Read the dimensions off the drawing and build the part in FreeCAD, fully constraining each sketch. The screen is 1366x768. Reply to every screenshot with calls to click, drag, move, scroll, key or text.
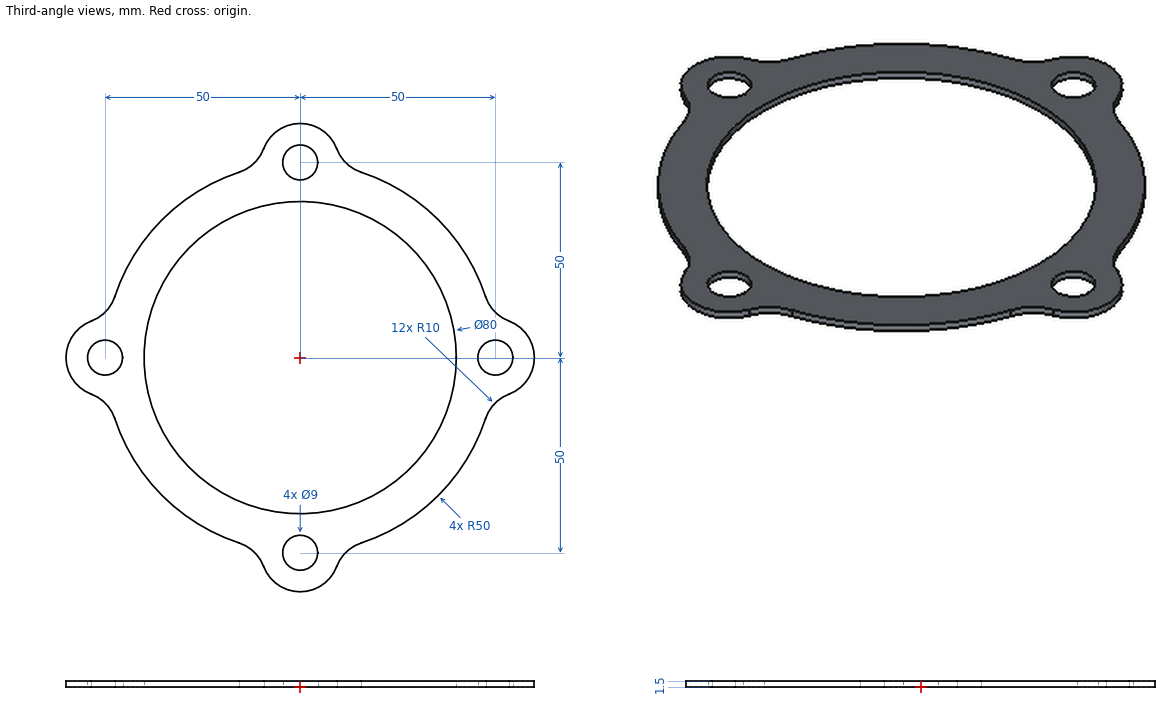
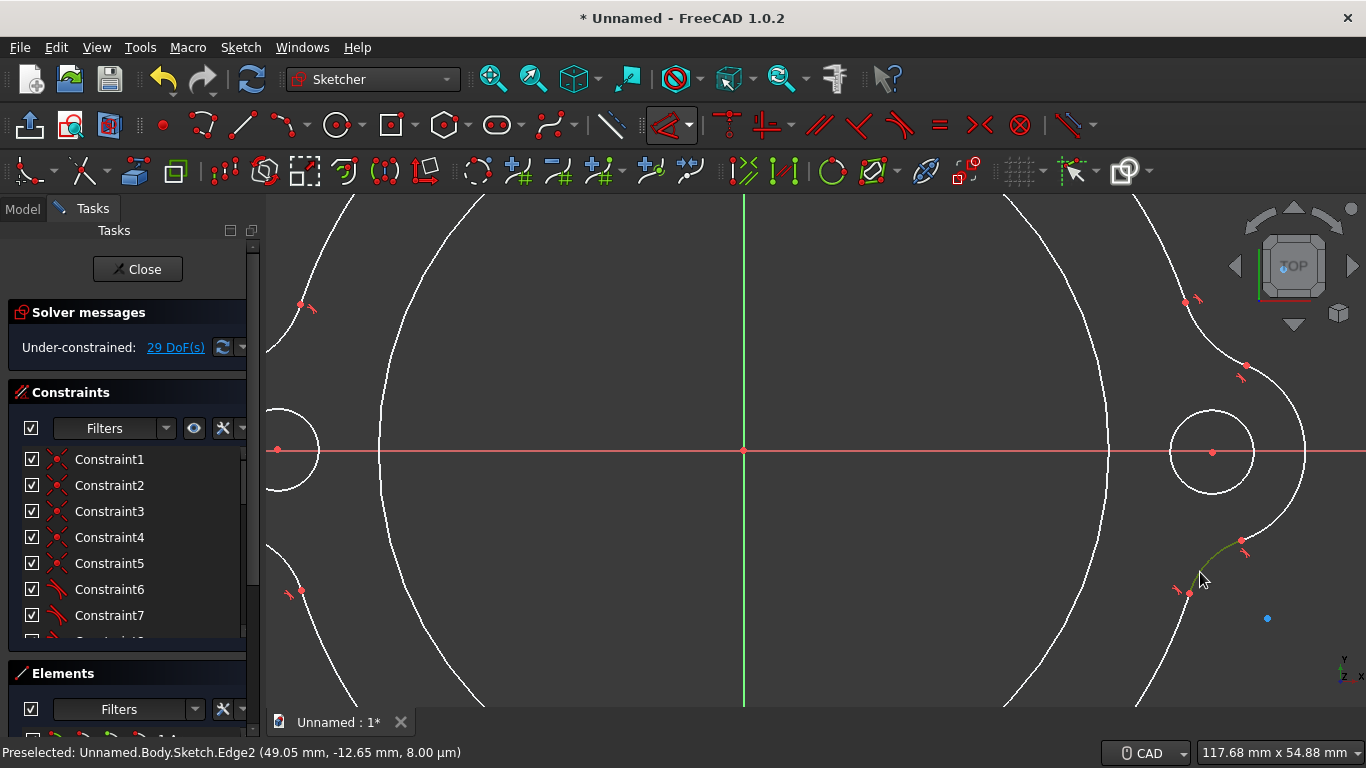
scroll(749, 450, down, 6)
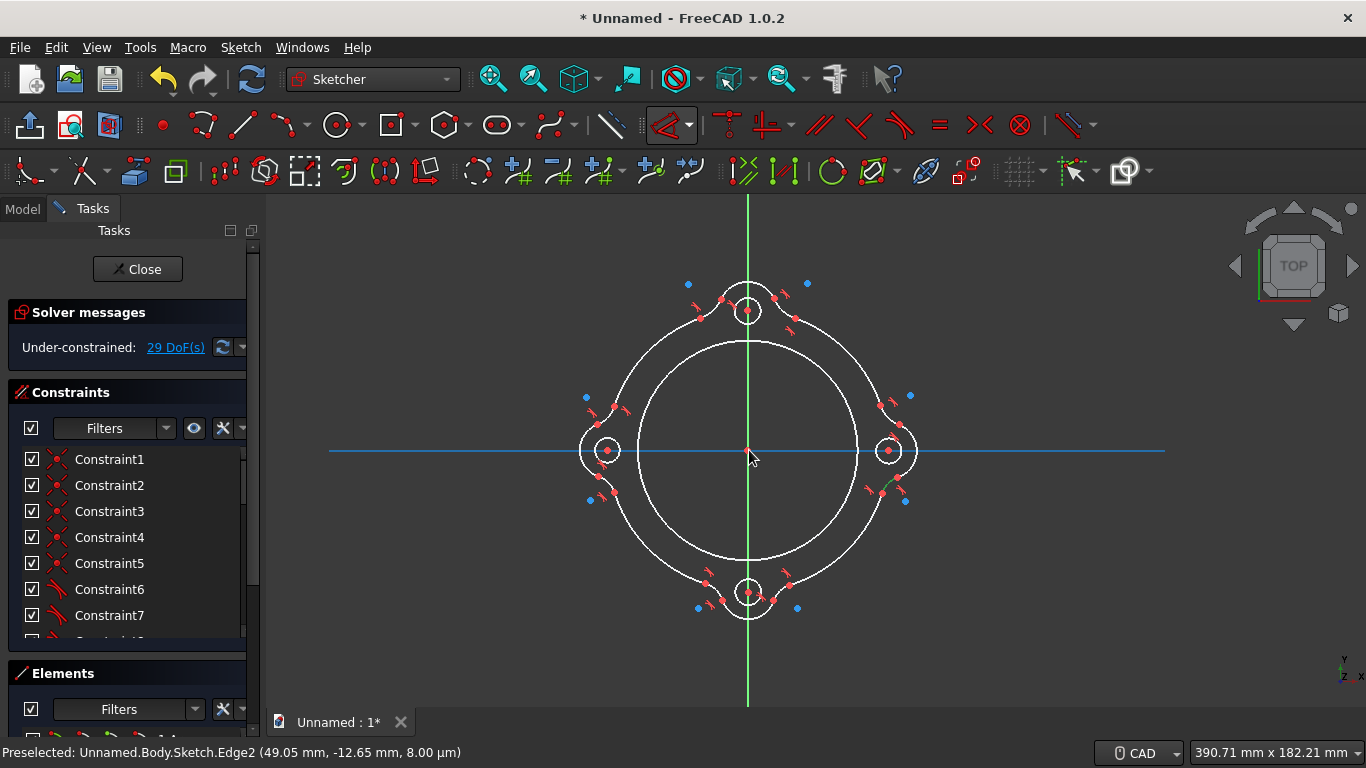
click(913, 465)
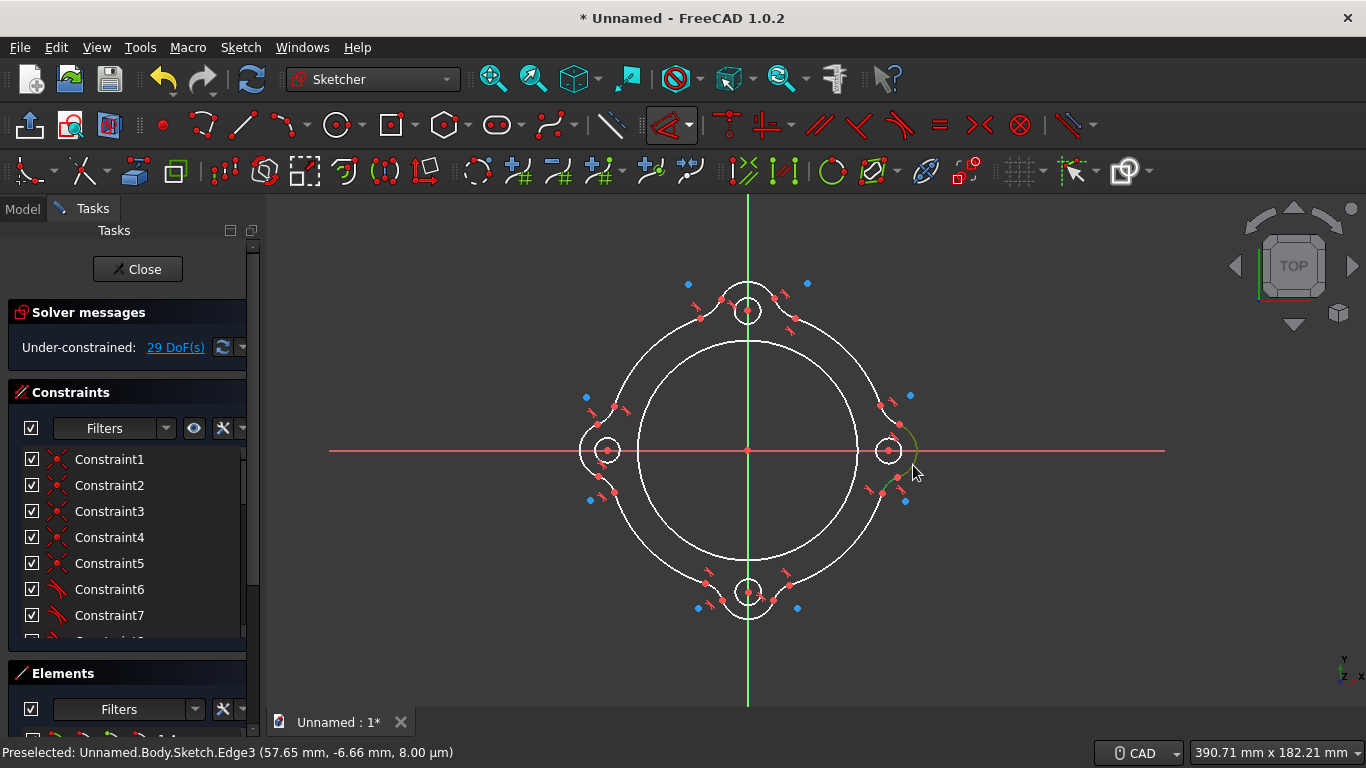
click(888, 417)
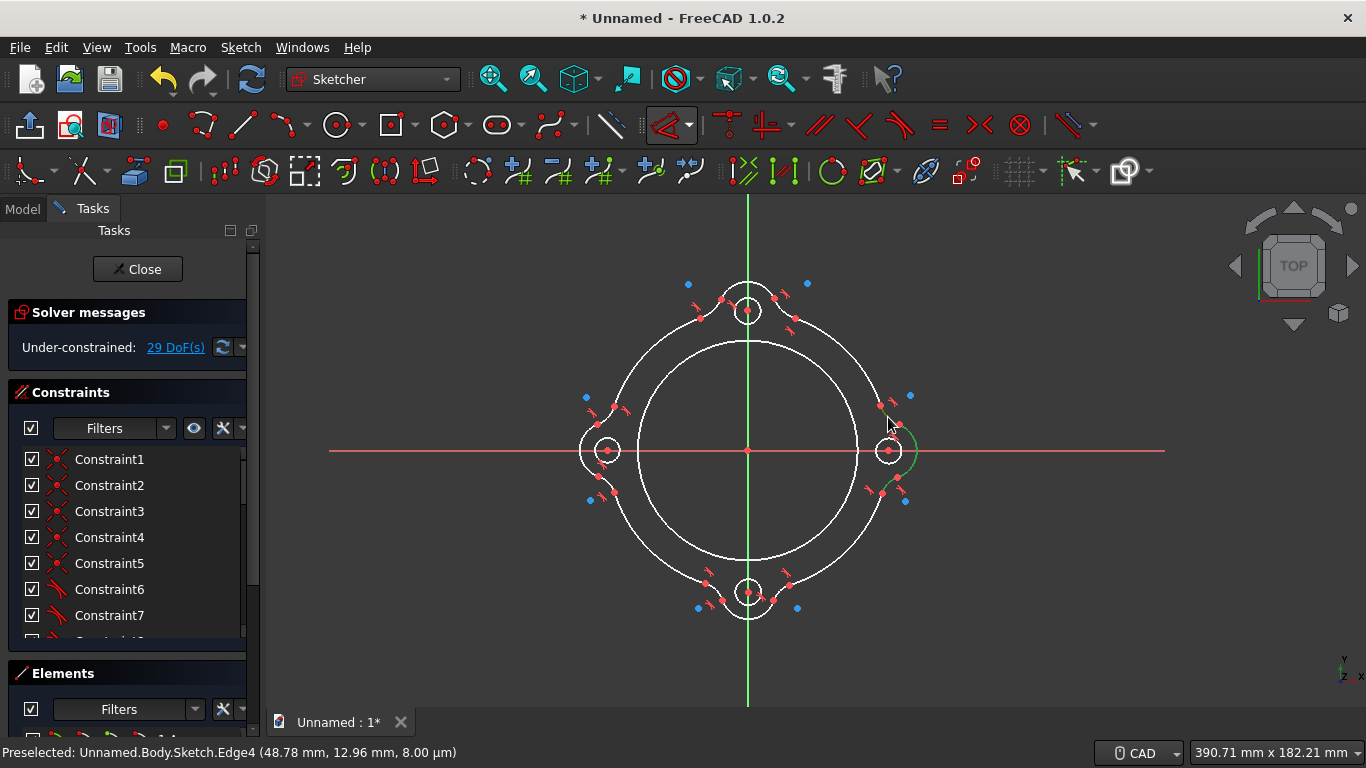
click(783, 311)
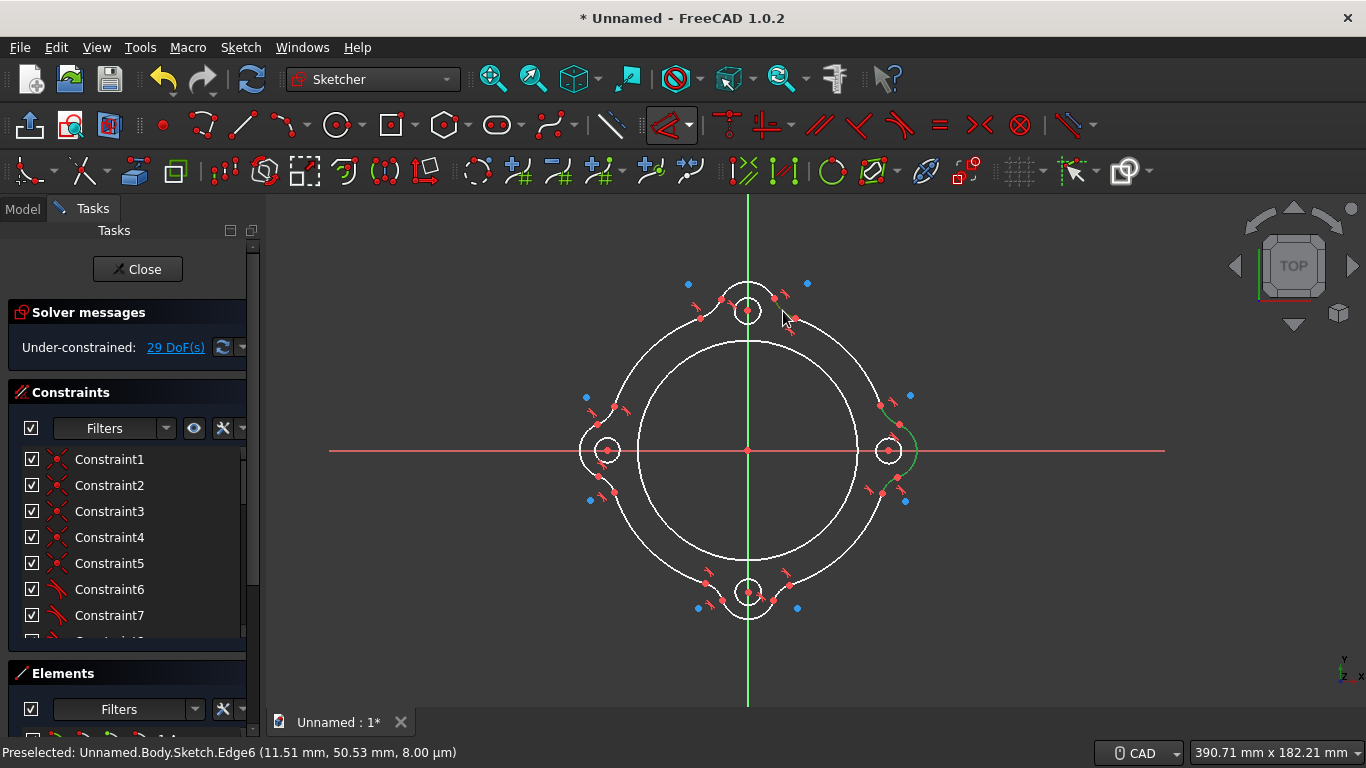
click(760, 285)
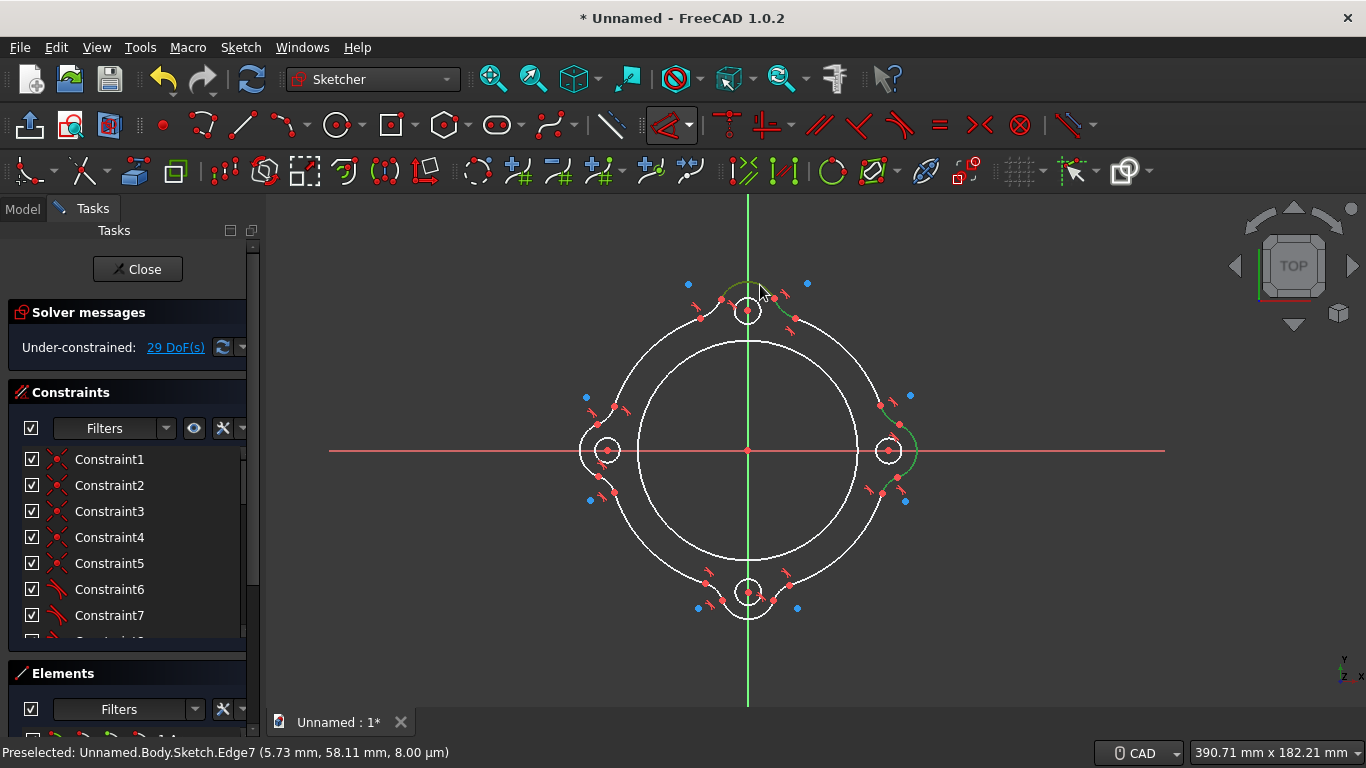
click(713, 311)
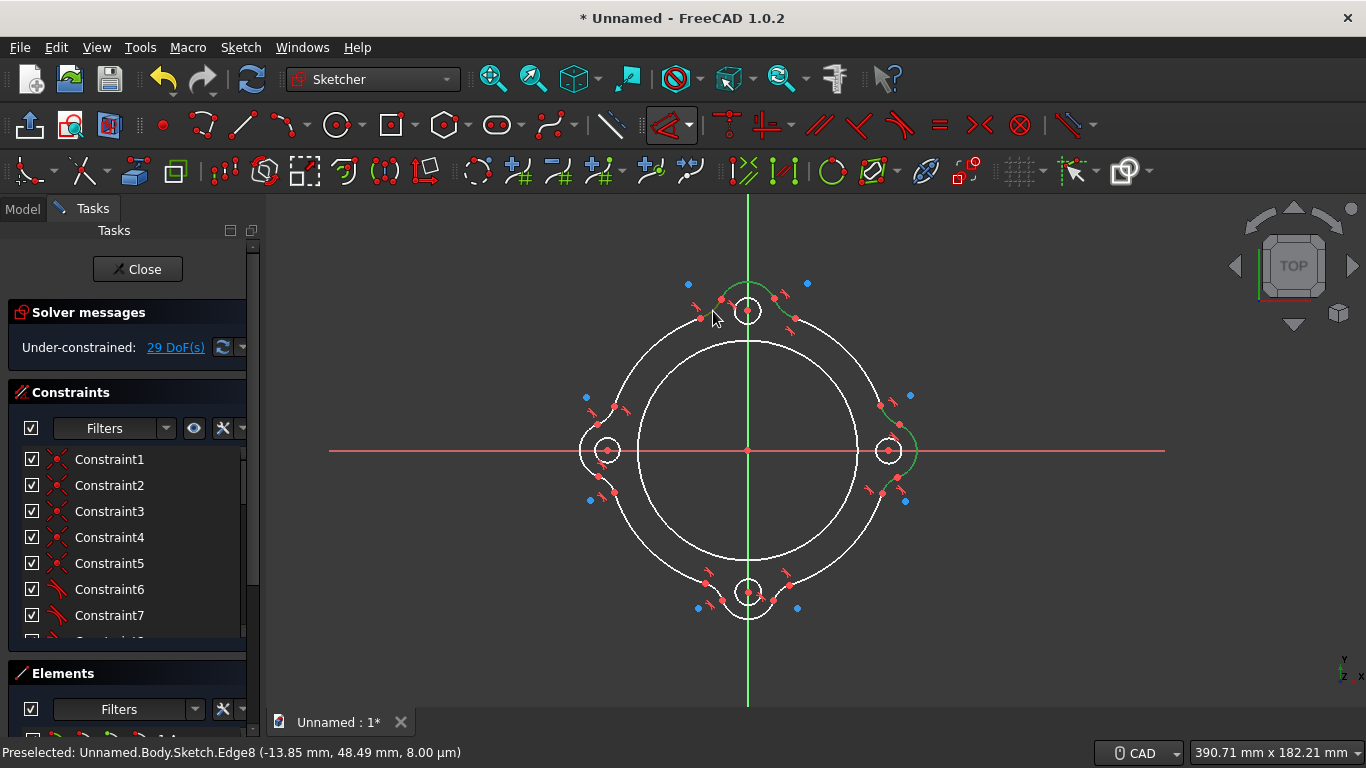
click(608, 418)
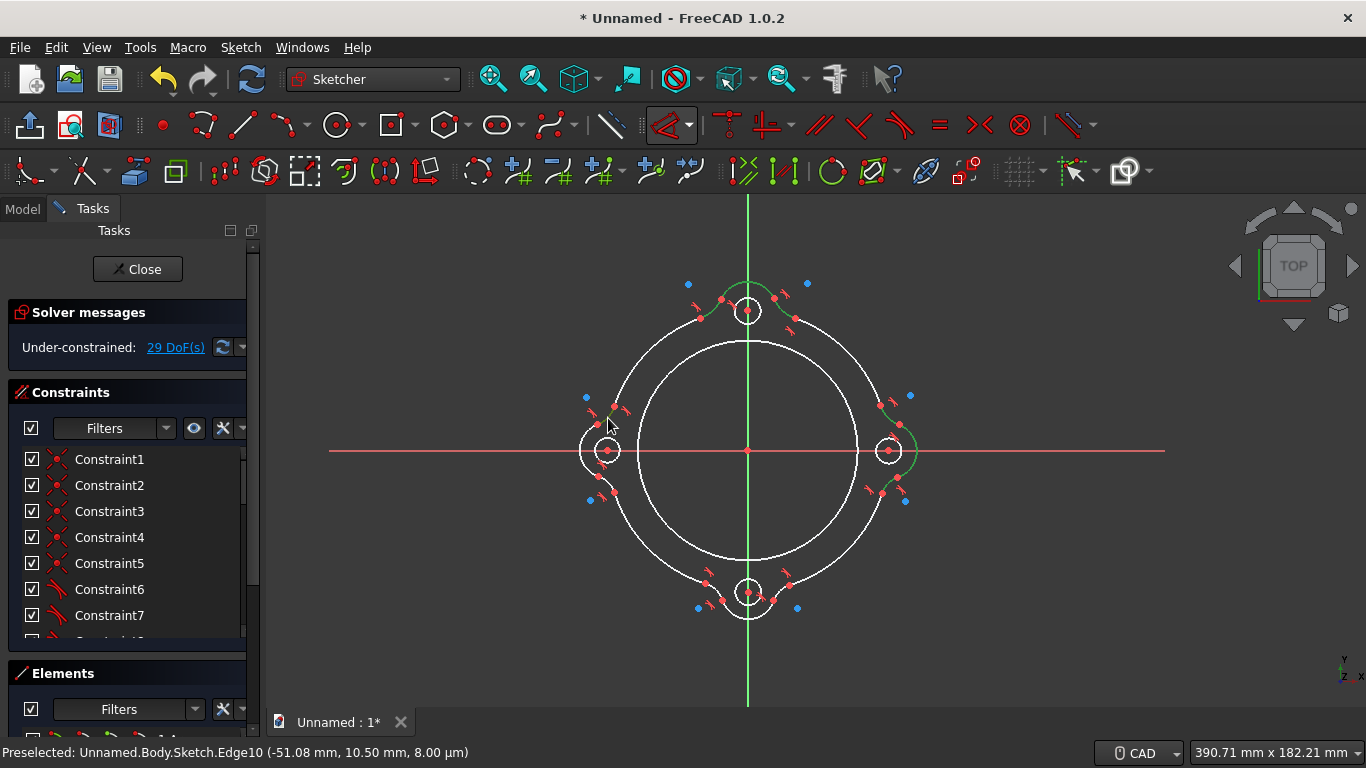
click(583, 438)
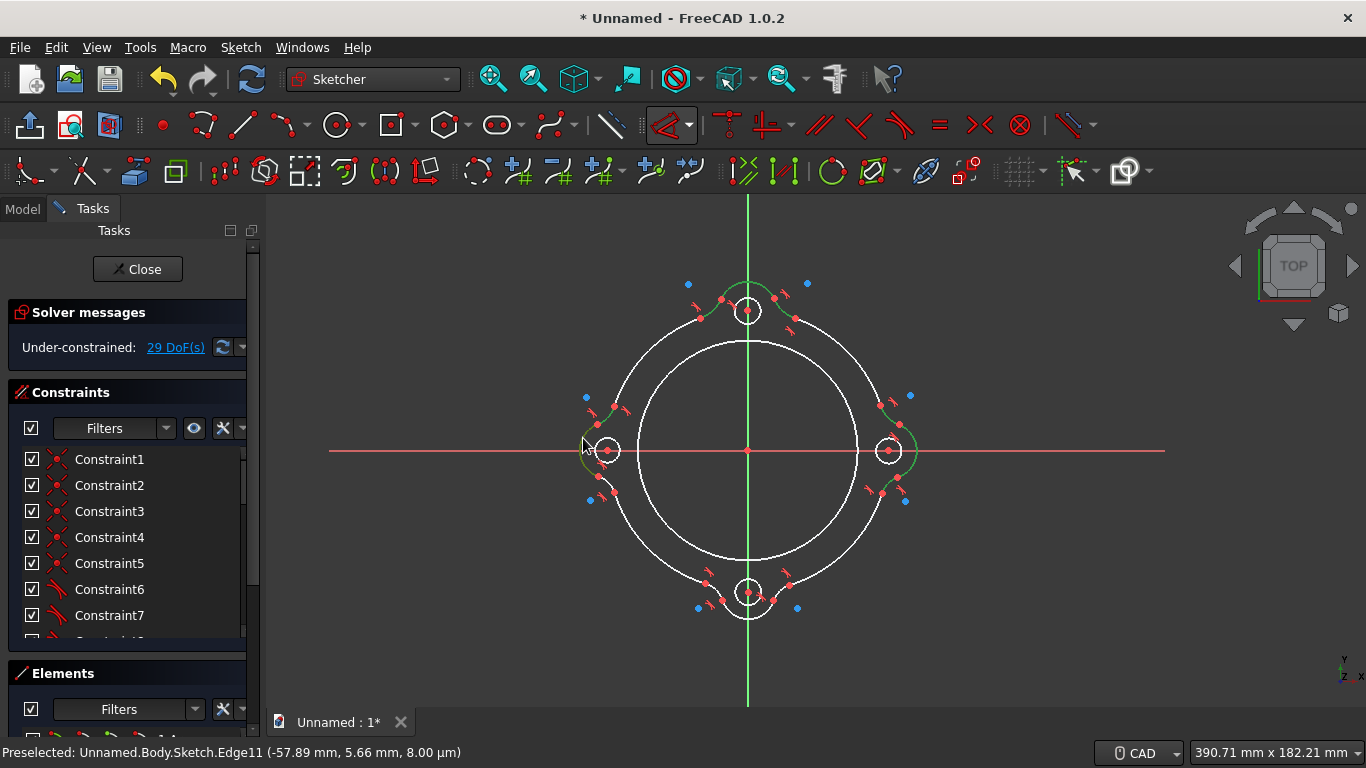
click(608, 483)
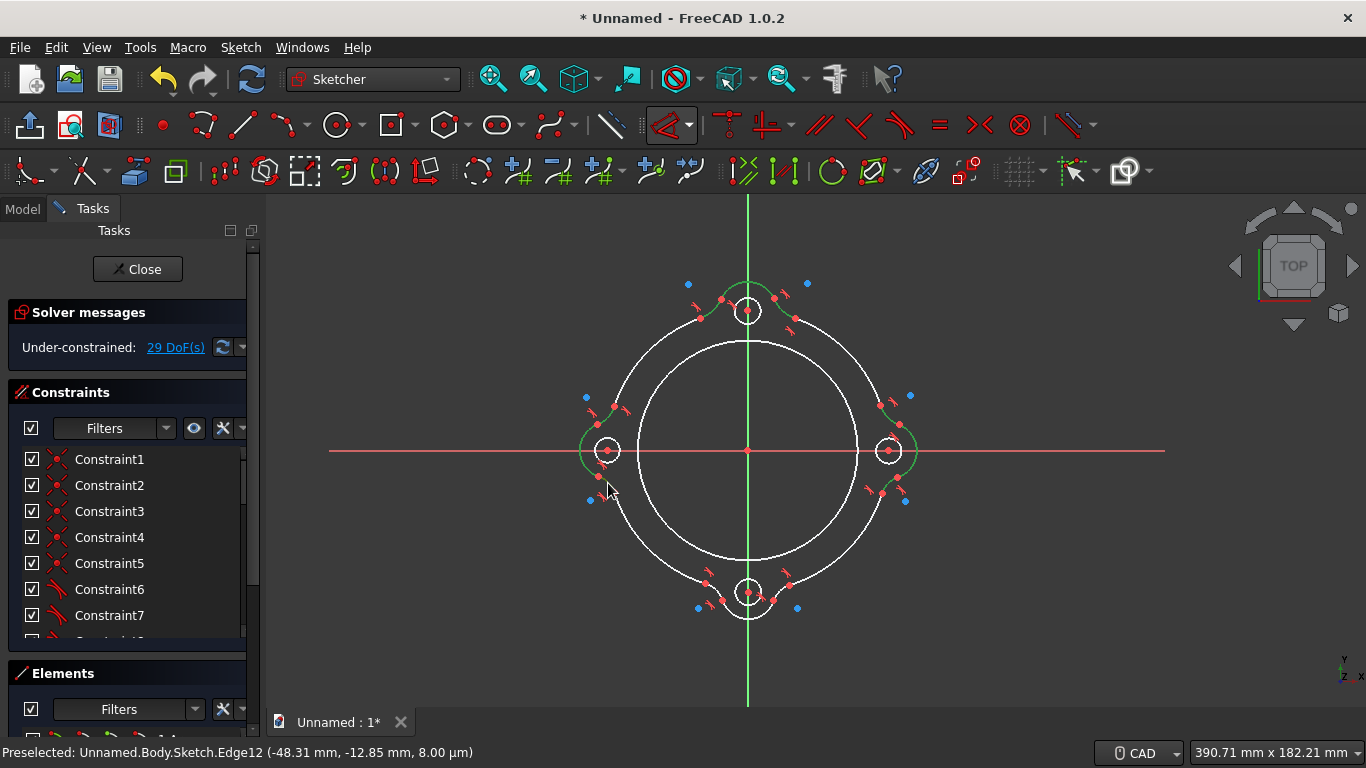
click(716, 590)